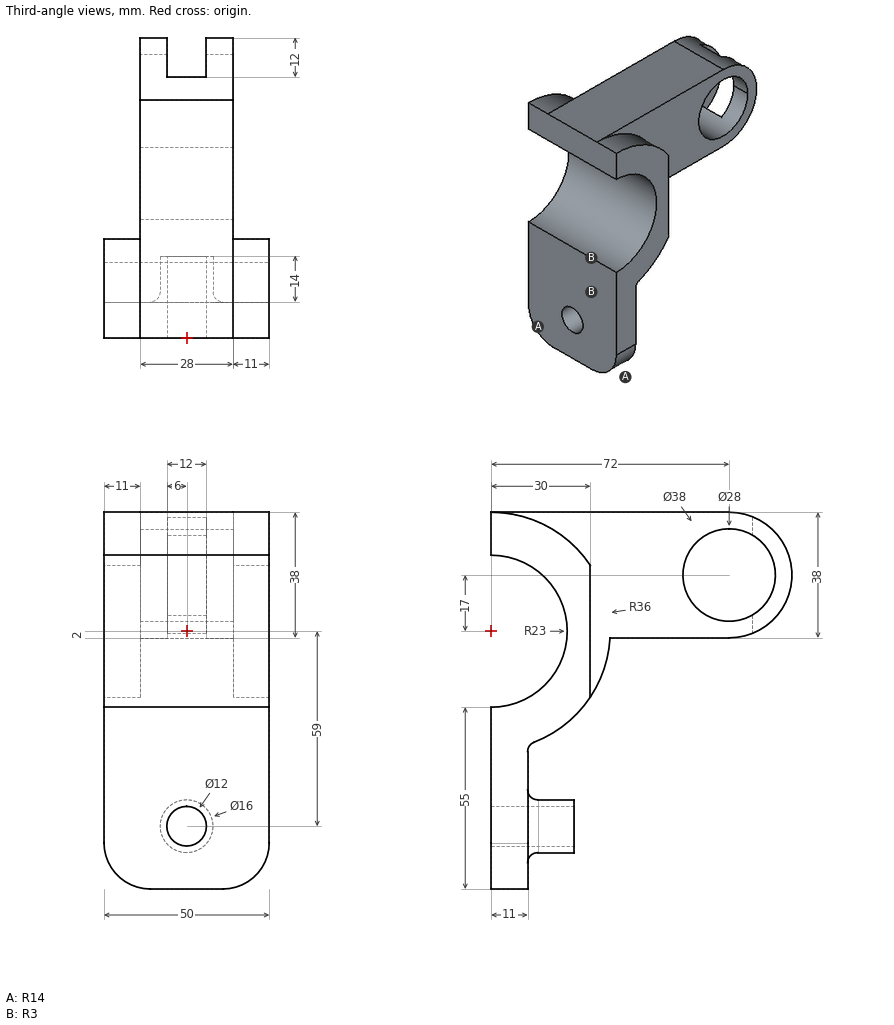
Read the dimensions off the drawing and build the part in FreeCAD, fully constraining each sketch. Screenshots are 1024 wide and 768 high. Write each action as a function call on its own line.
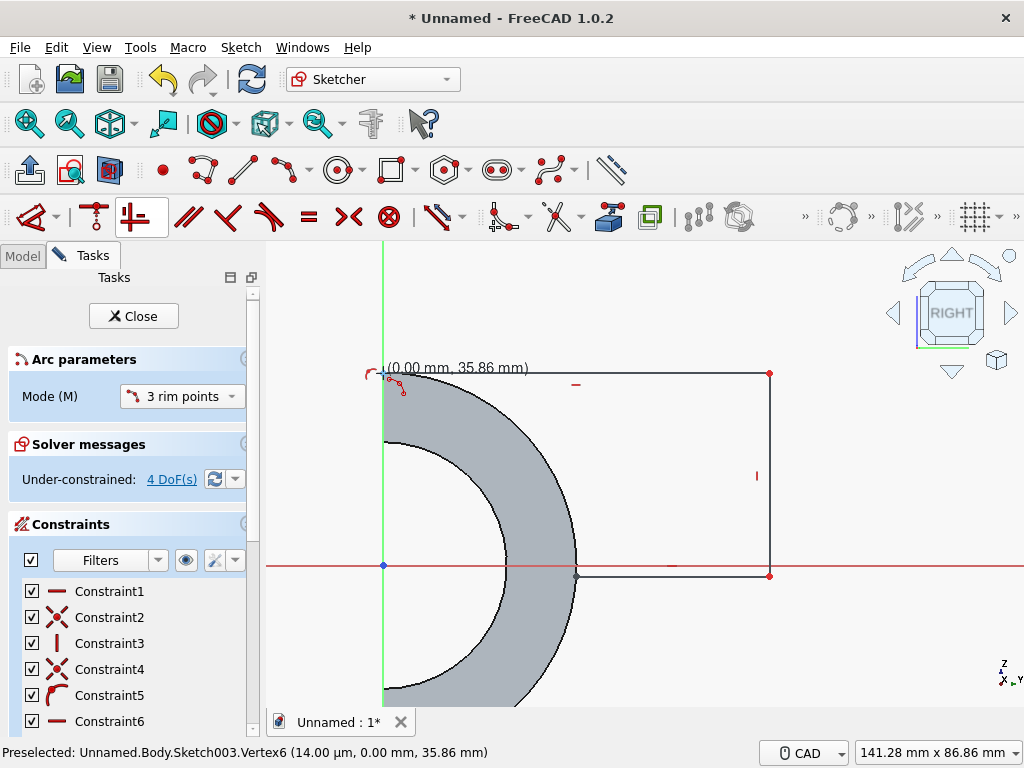
scroll(576, 576, up, 2)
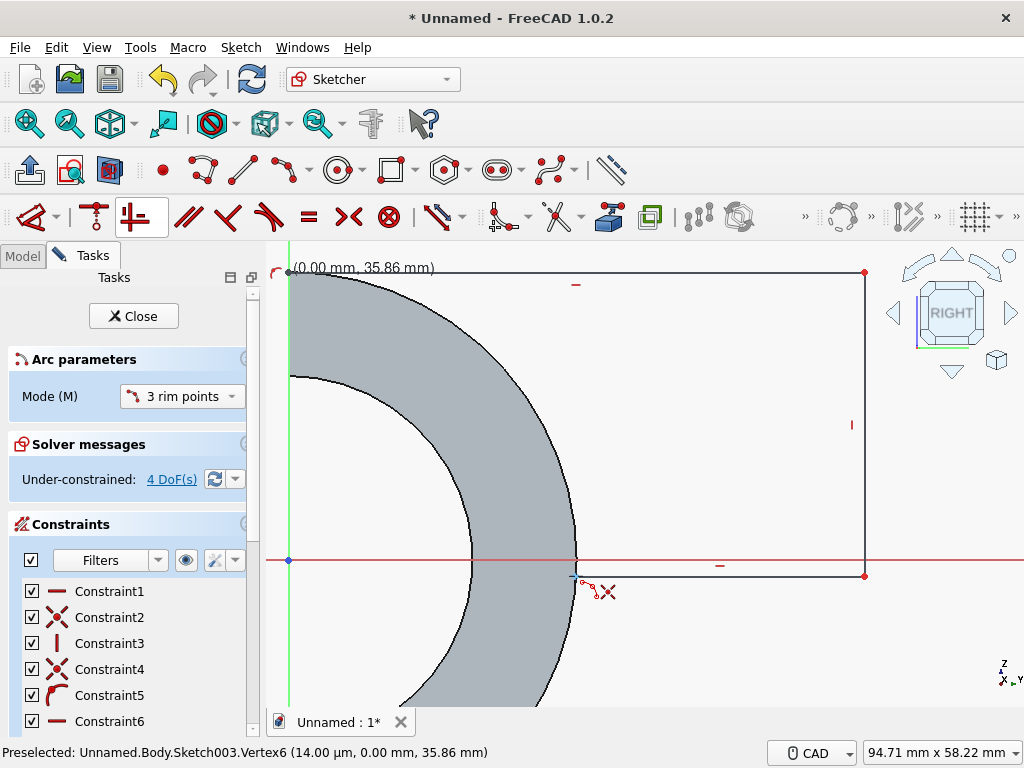
click(576, 577)
click(498, 362)
key(Escape)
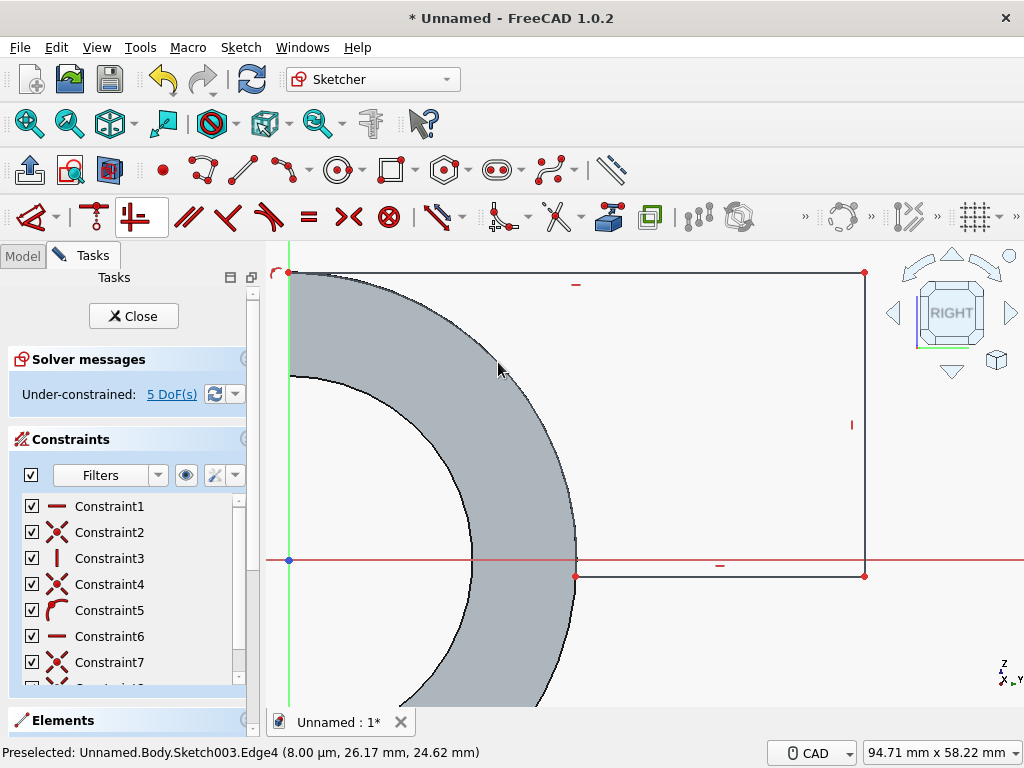
scroll(576, 576, down, 2)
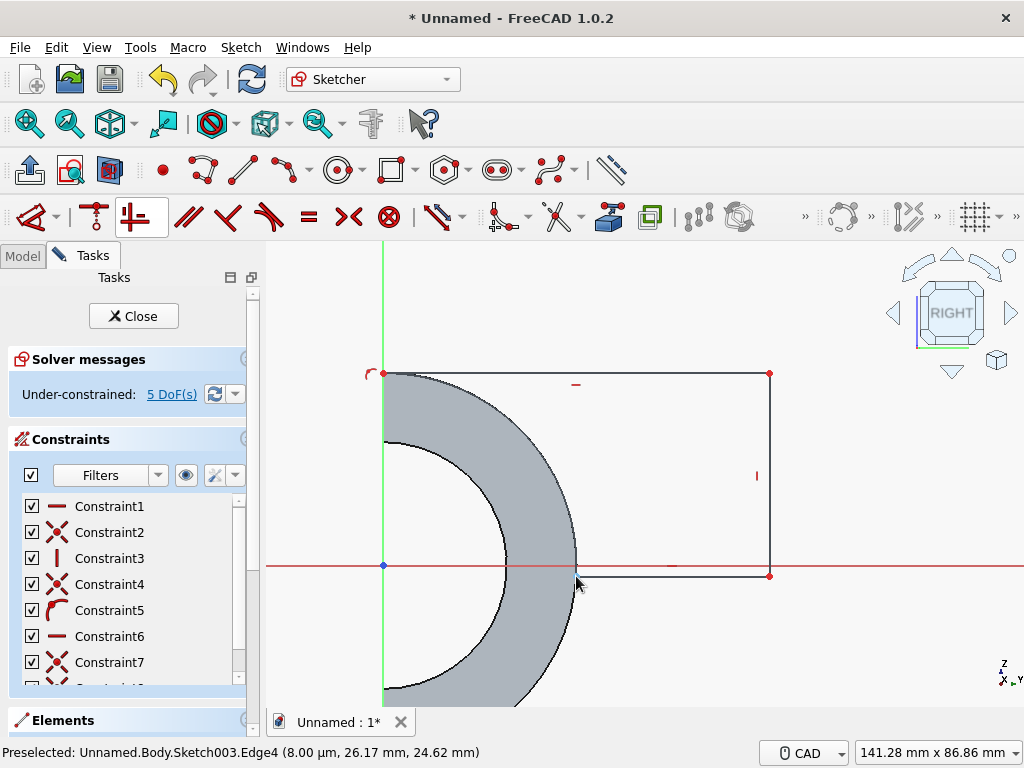
drag(373, 556, 394, 576)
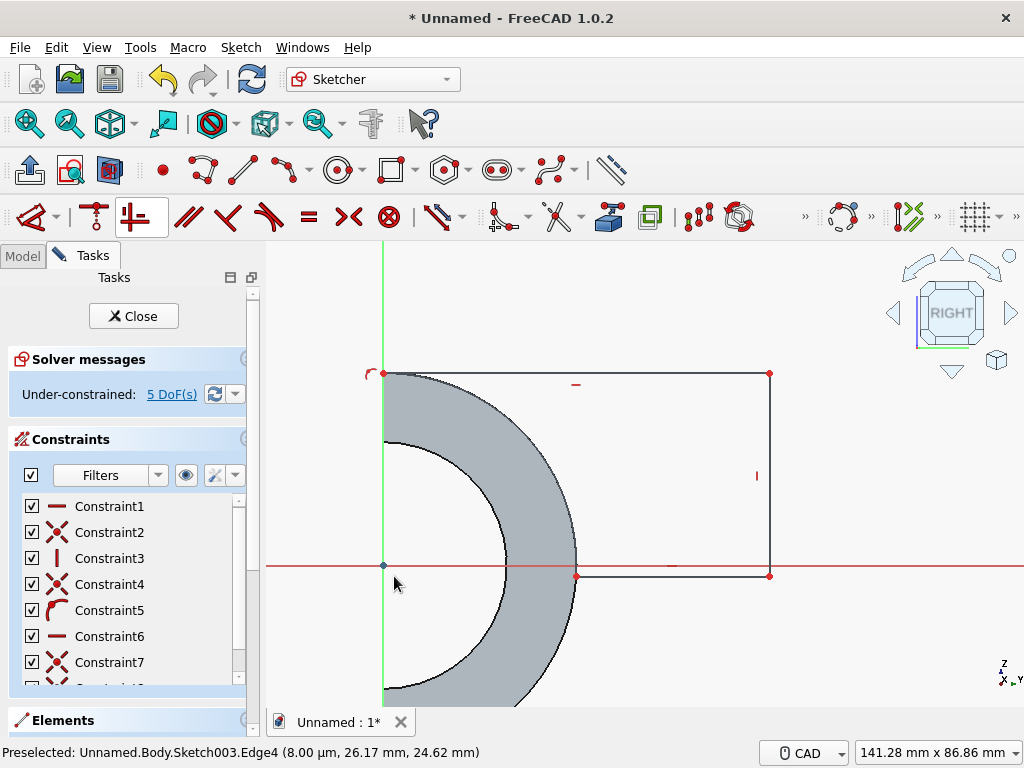
click(94, 218)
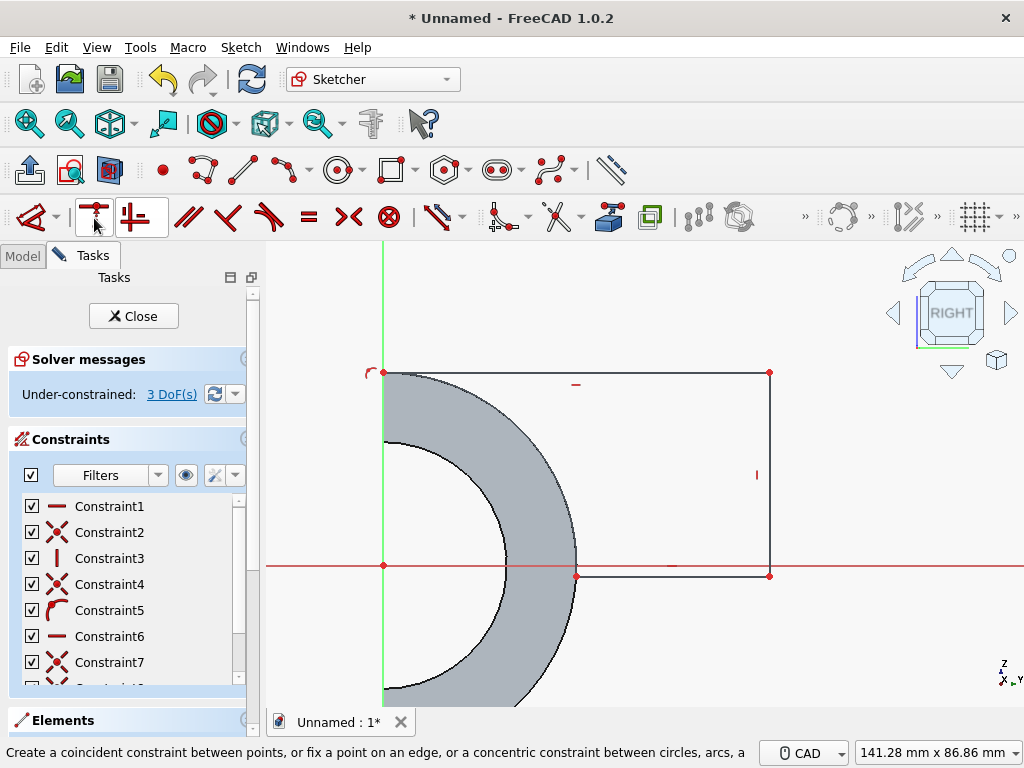
click(32, 218)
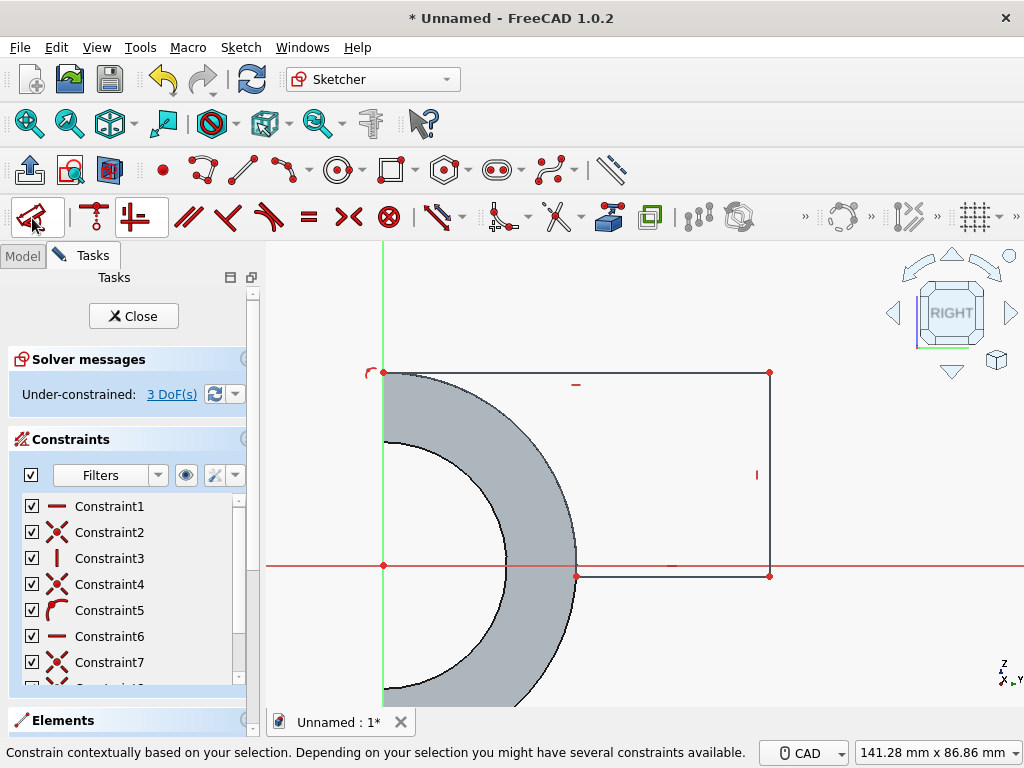
click(559, 485)
click(588, 472)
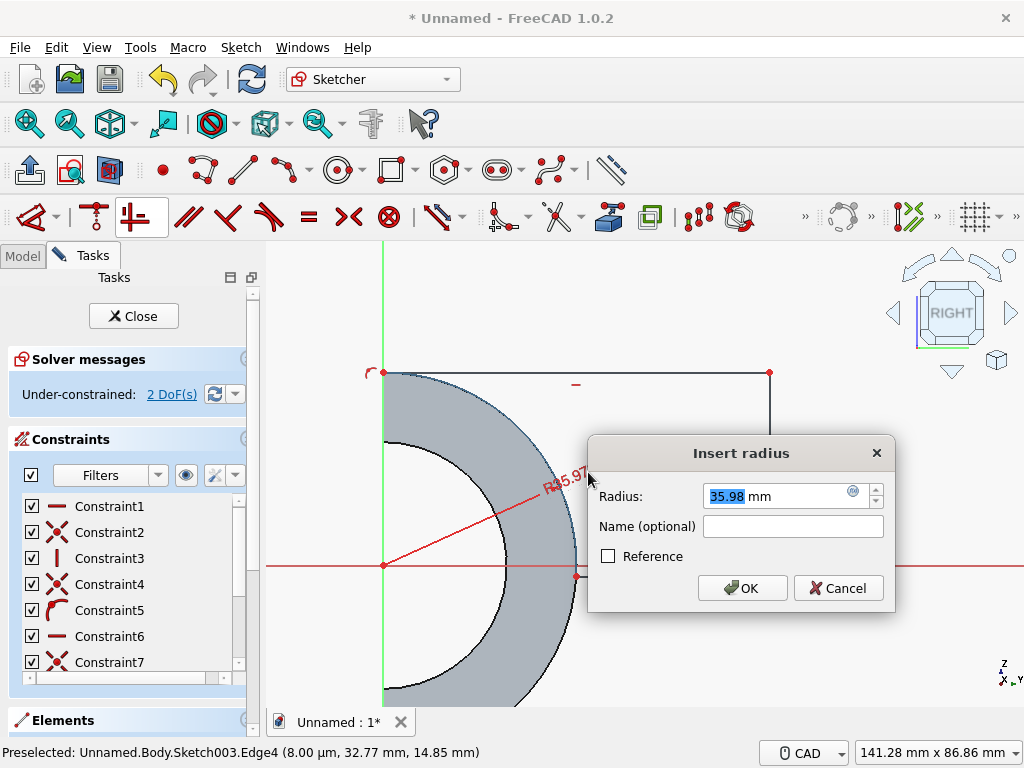
text(36)
key(Return)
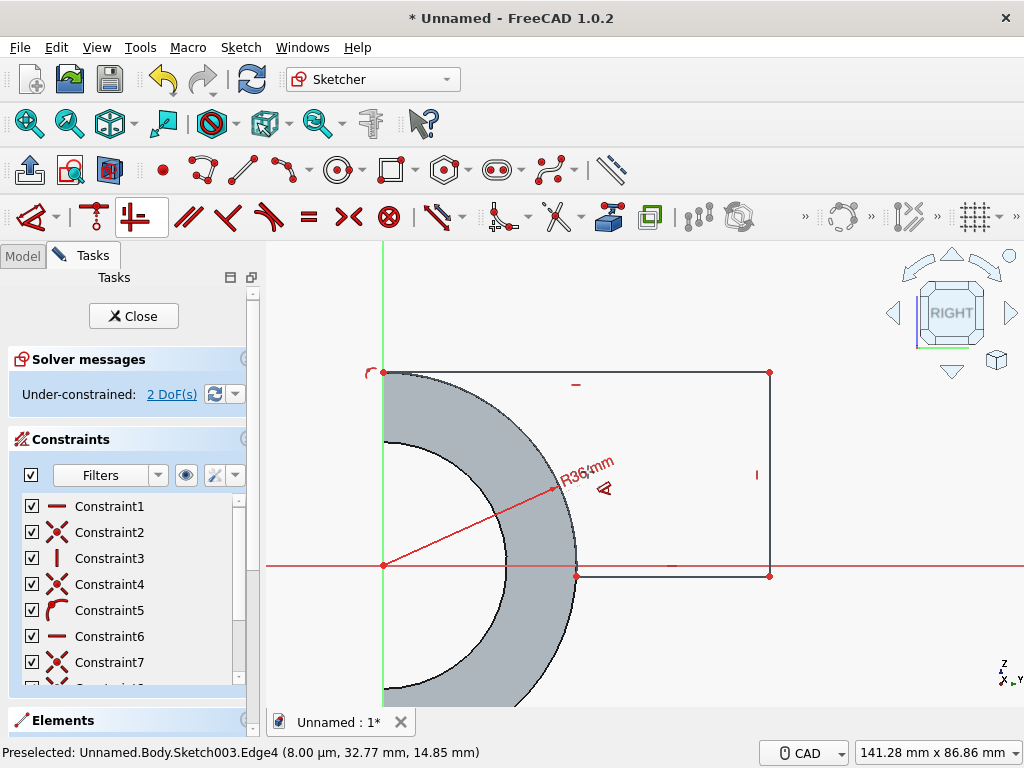
click(770, 516)
click(804, 475)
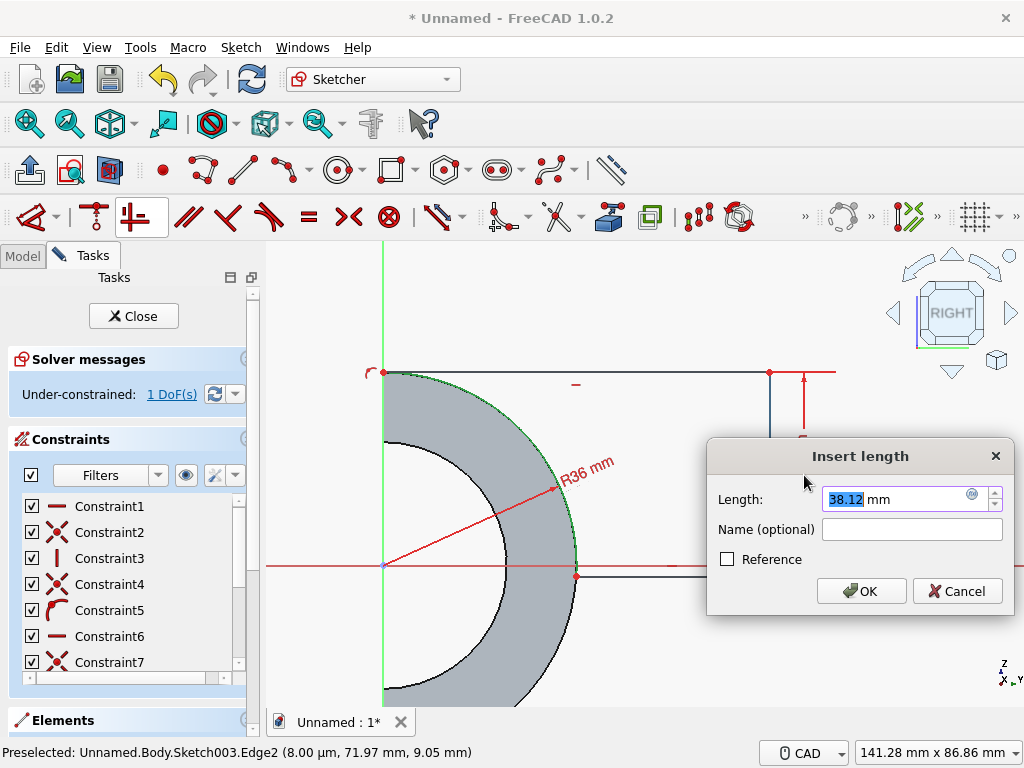
text(38)
key(Return)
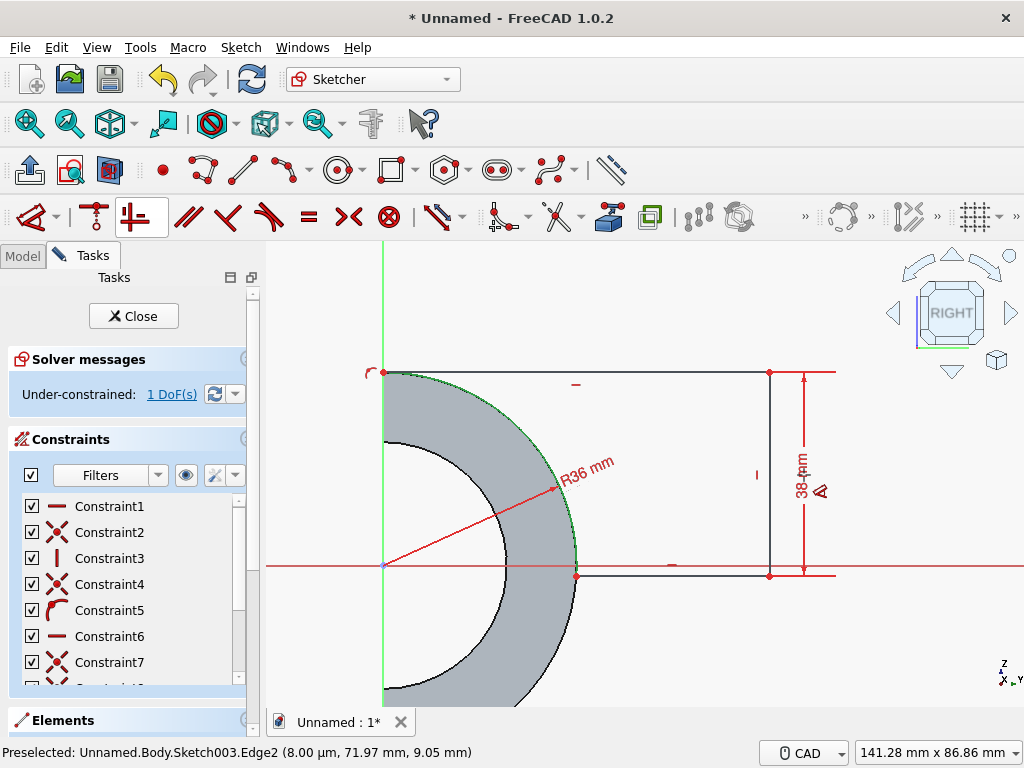
click(654, 372)
click(576, 338)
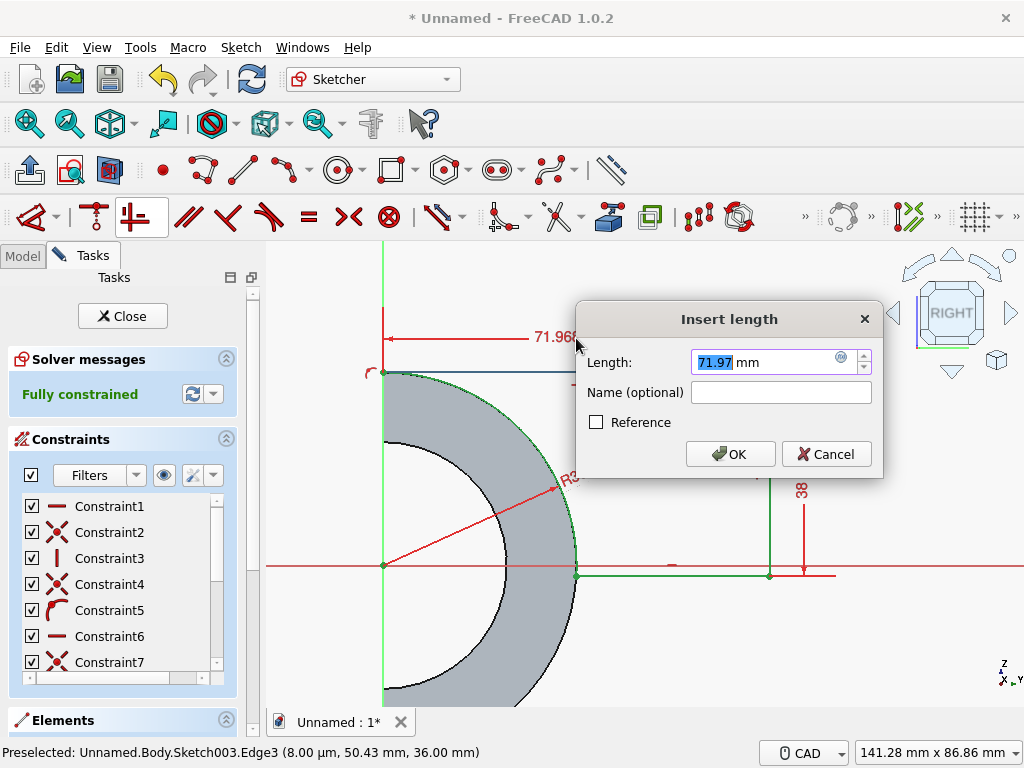
text(72)
key(Return)
key(Escape)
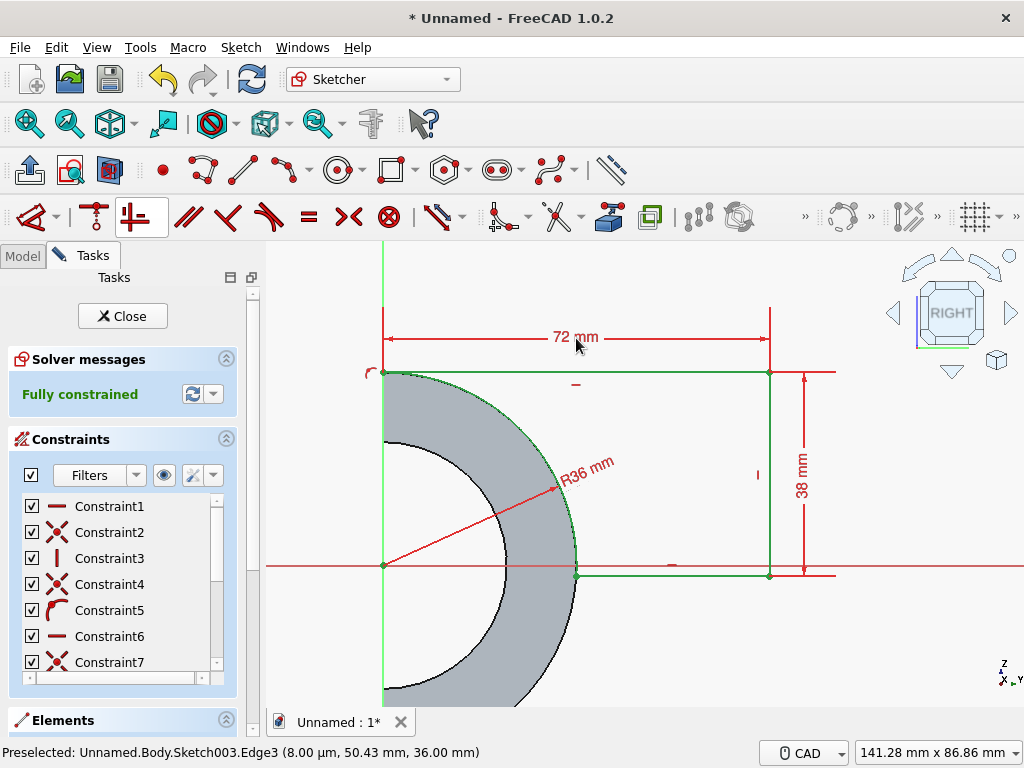
click(123, 316)